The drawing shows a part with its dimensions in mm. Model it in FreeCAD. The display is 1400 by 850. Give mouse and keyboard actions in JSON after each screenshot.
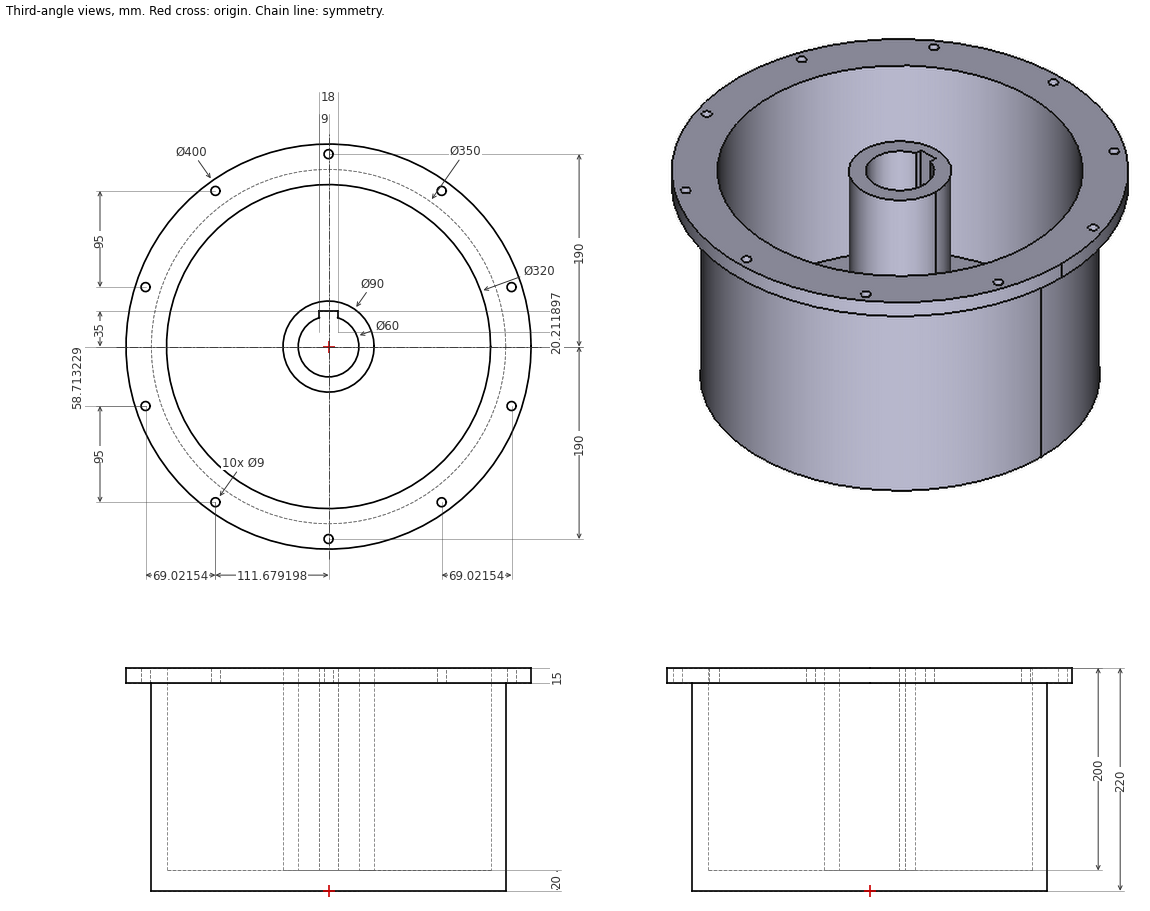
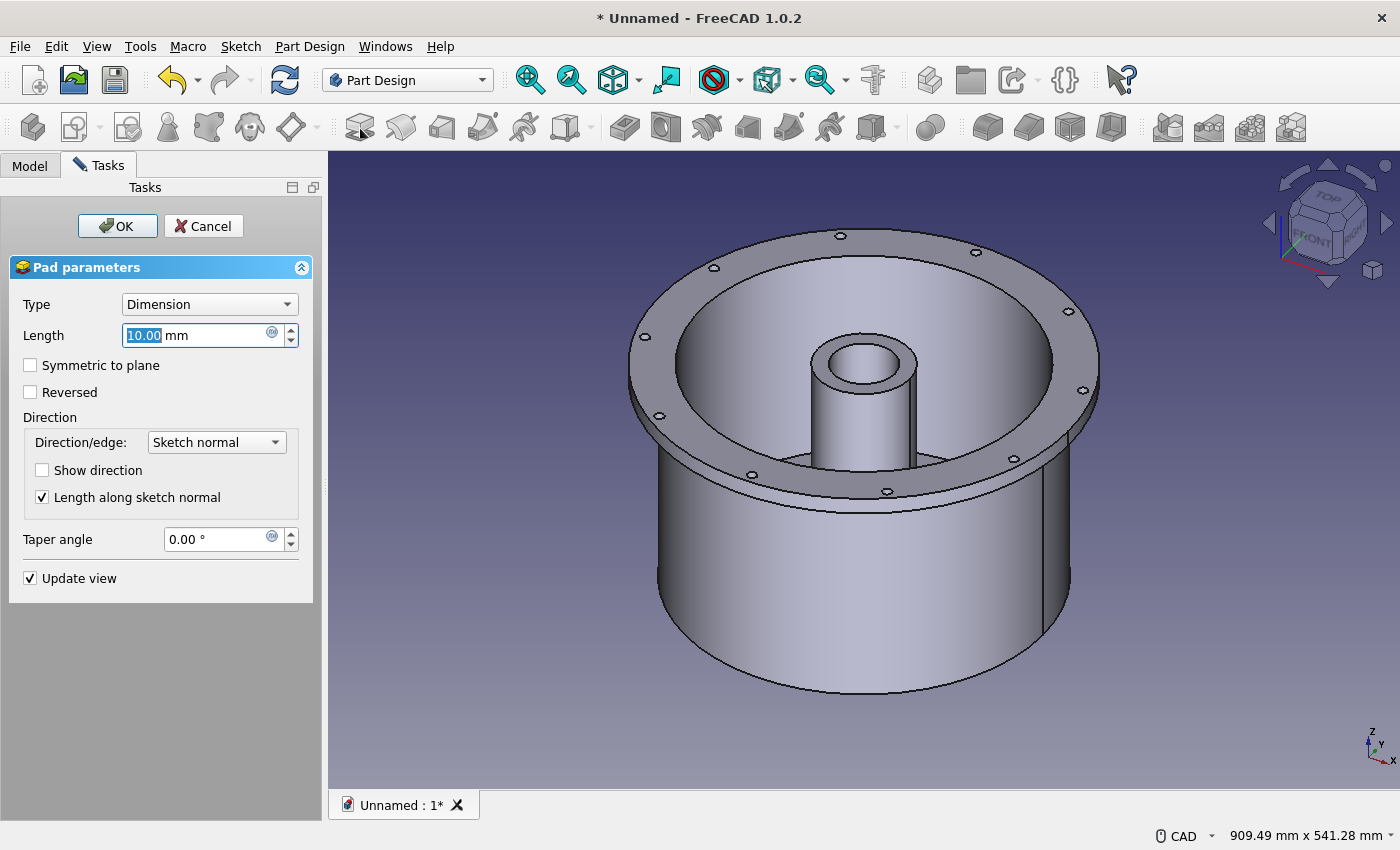
{"action": "type", "text": "20"}
{"action": "key", "text": "Tab"}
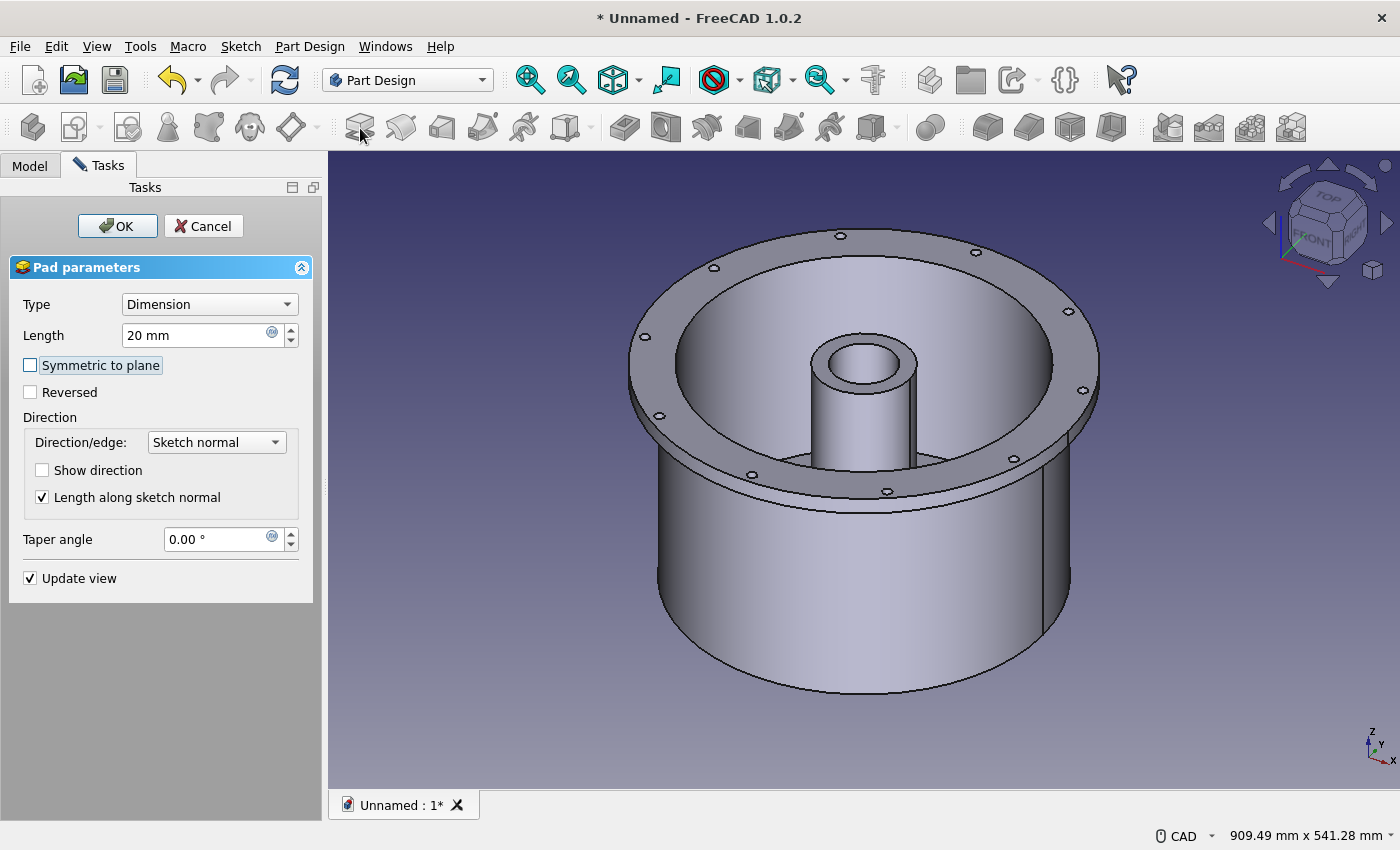
{"action": "left_click", "coordinate": [118, 226]}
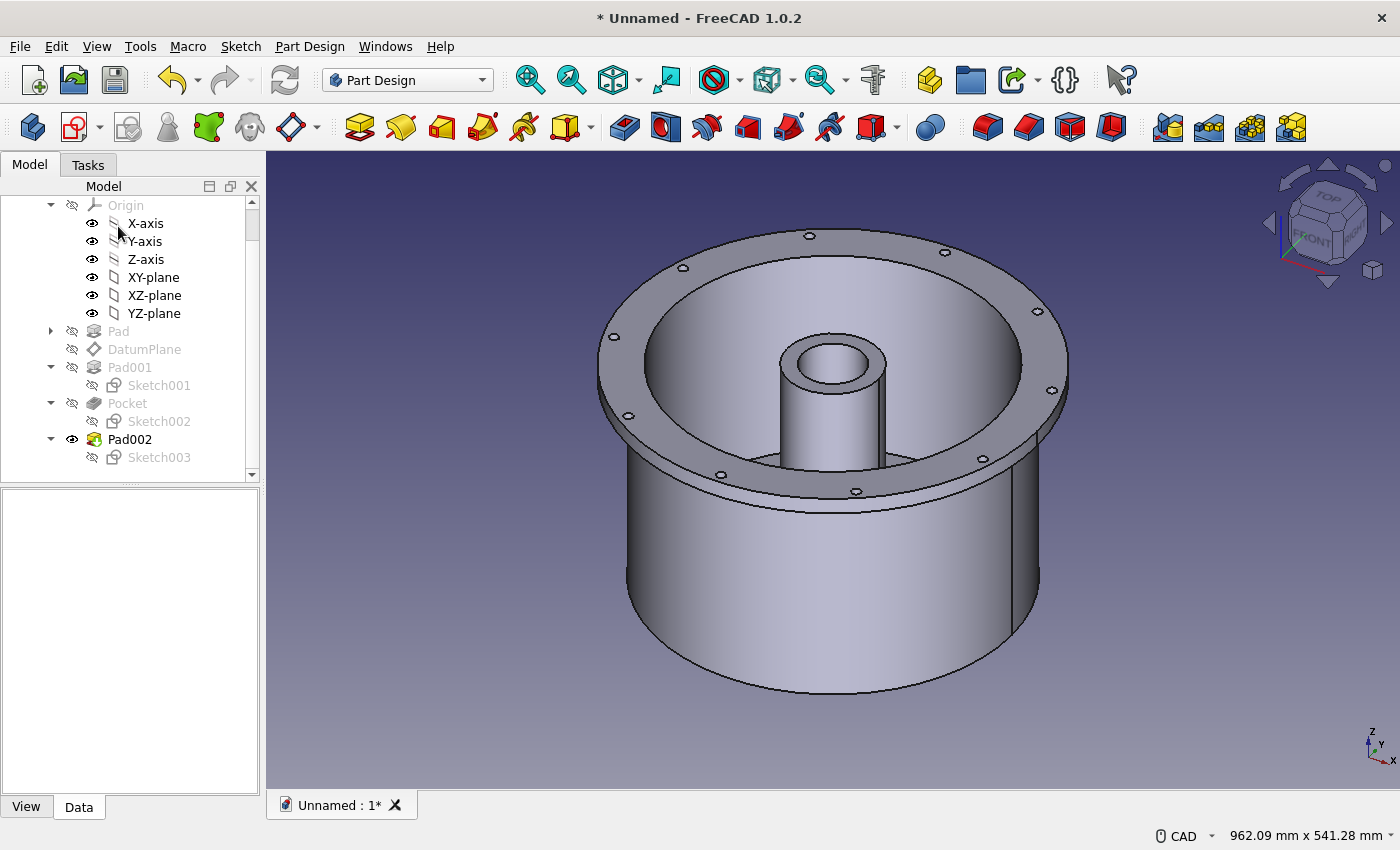
{"action": "left_click", "coordinate": [790, 482]}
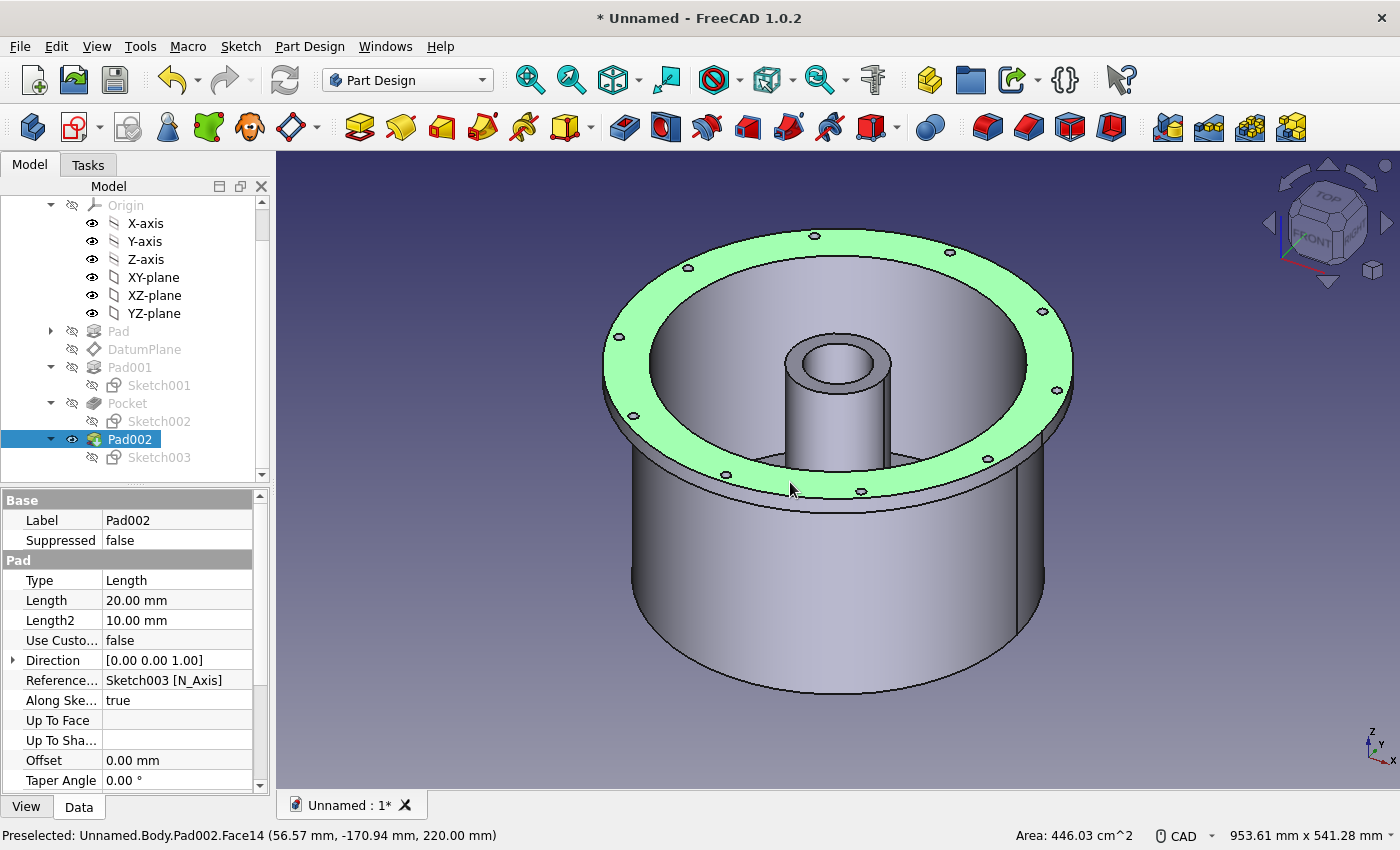
{"action": "left_click", "coordinate": [74, 128]}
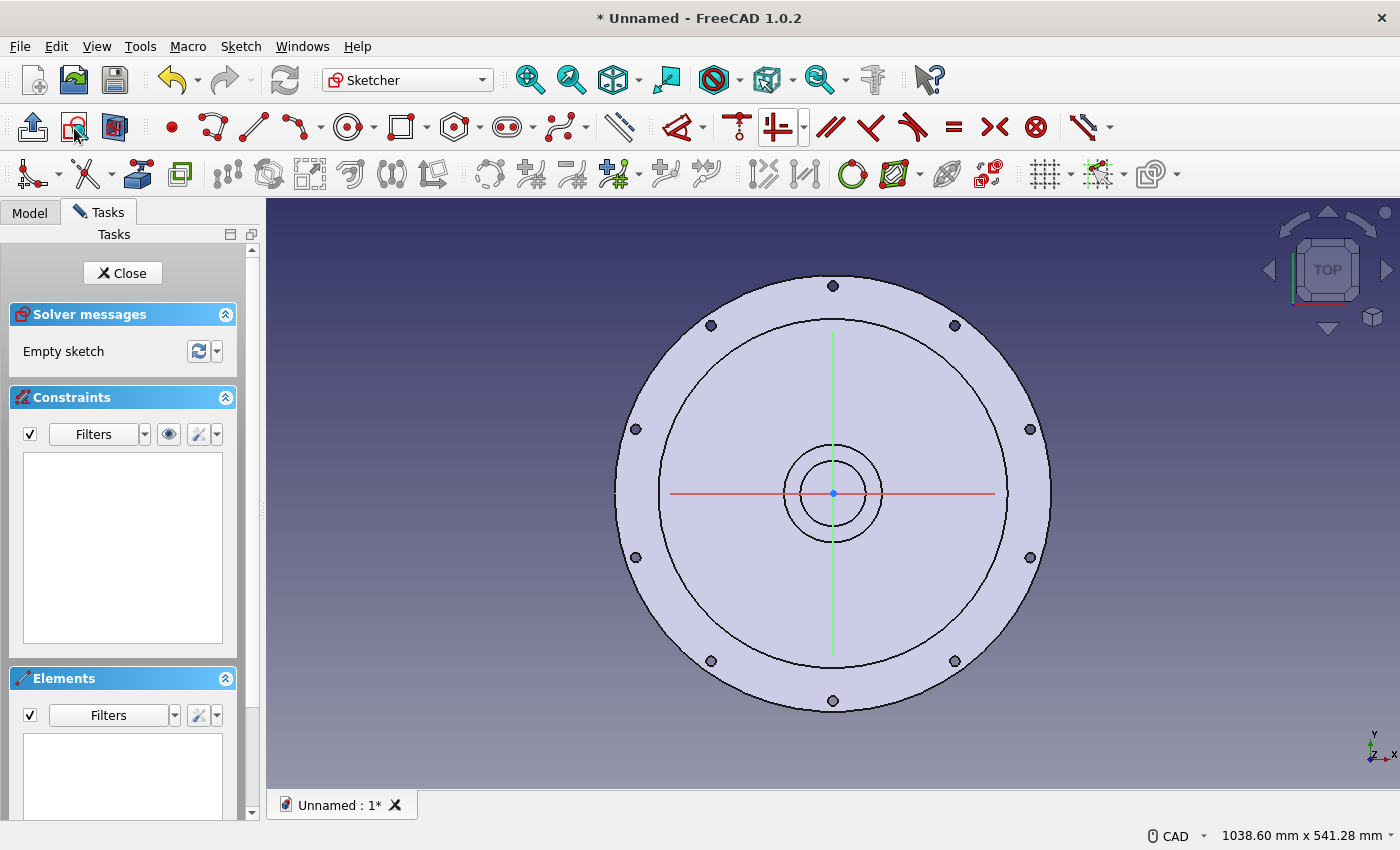
{"action": "scroll", "coordinate": [842, 472], "scroll_direction": "up", "scroll_amount": 11}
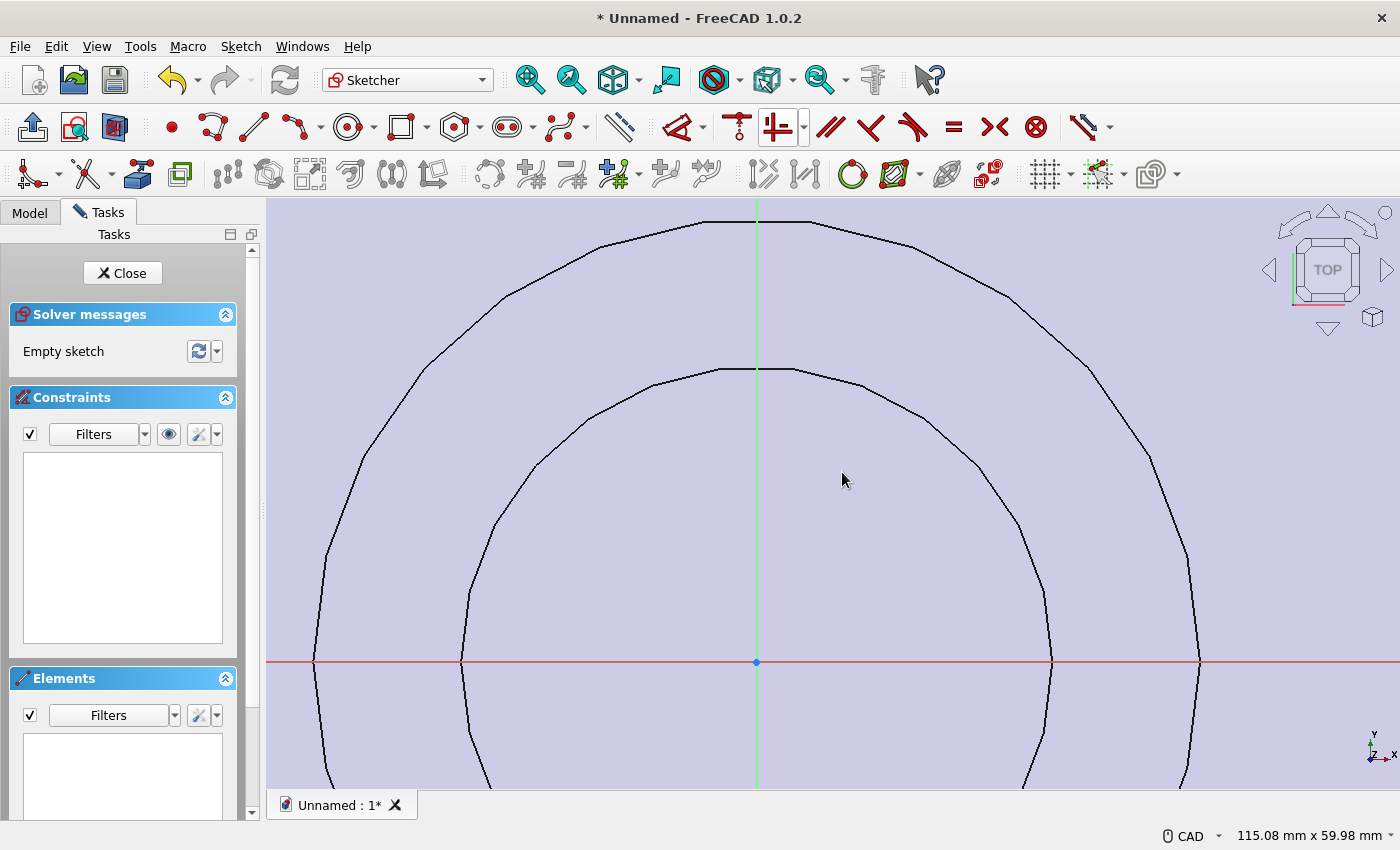
{"action": "left_click", "coordinate": [400, 128]}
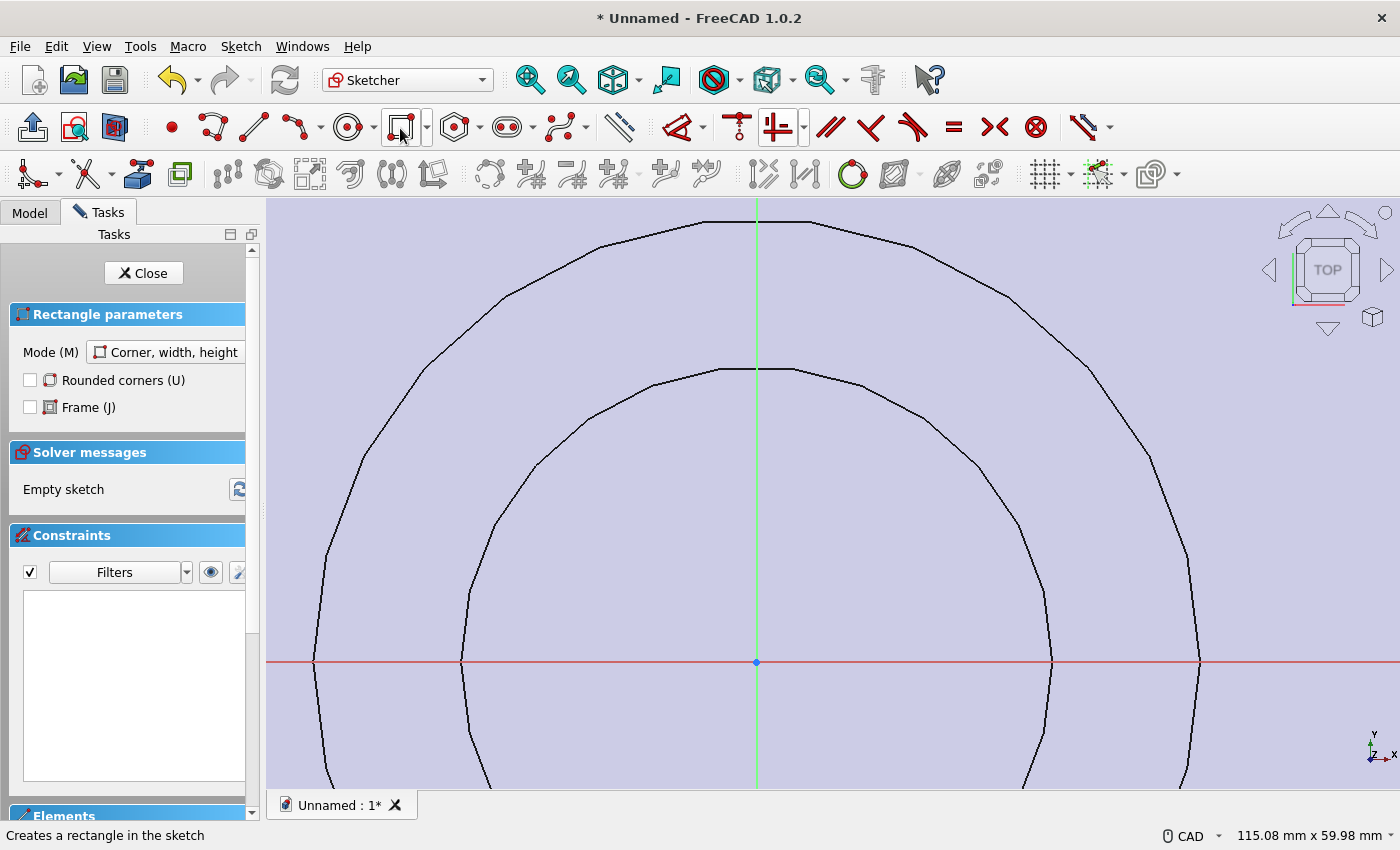
{"action": "left_click", "coordinate": [668, 317]}
{"action": "mouse_move", "coordinate": [845, 517]}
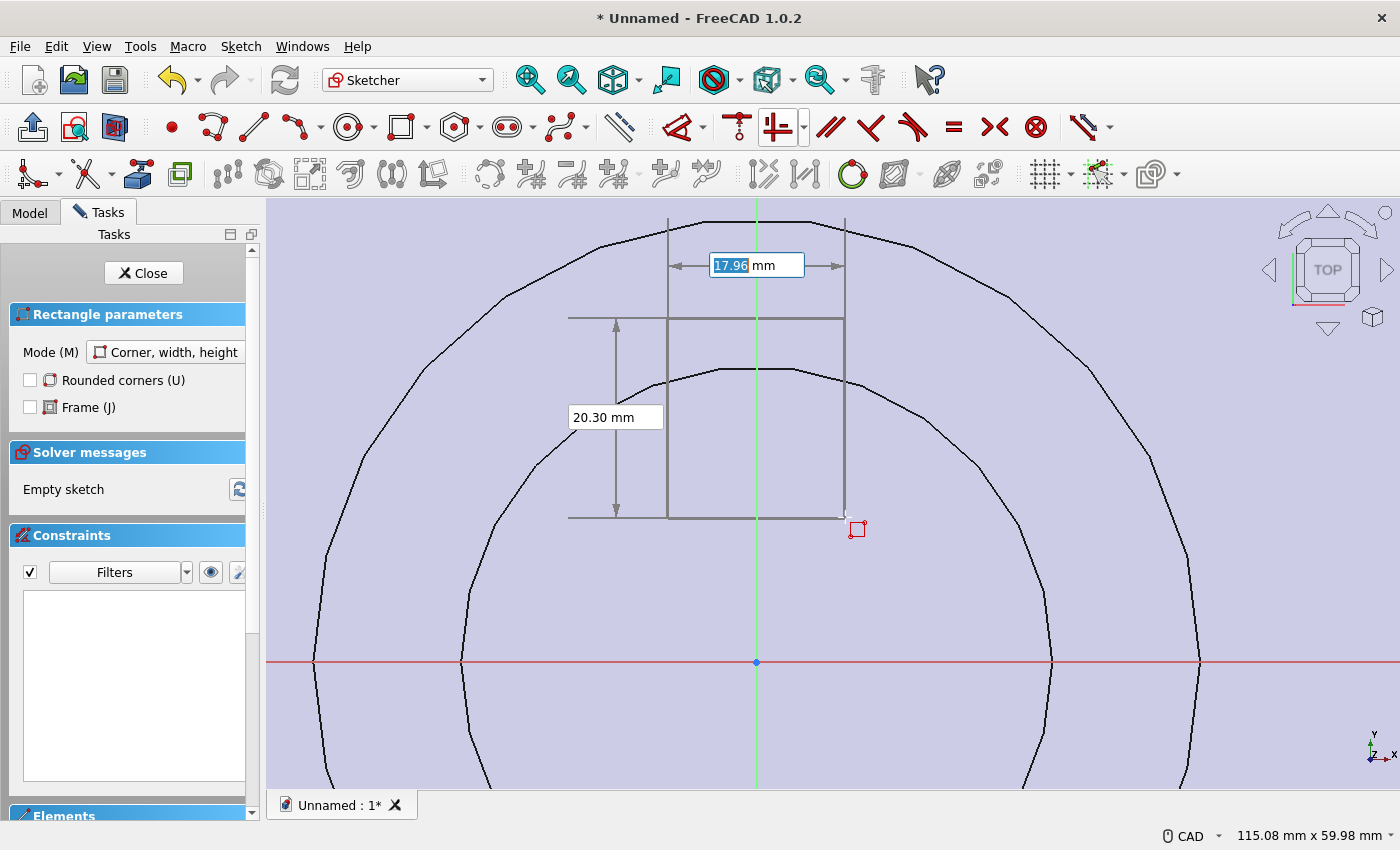
{"action": "type", "text": "18"}
{"action": "key", "text": "Tab"}
{"action": "type", "text": "20.211897"}
{"action": "key", "text": "Return"}
{"action": "key", "text": "Escape"}